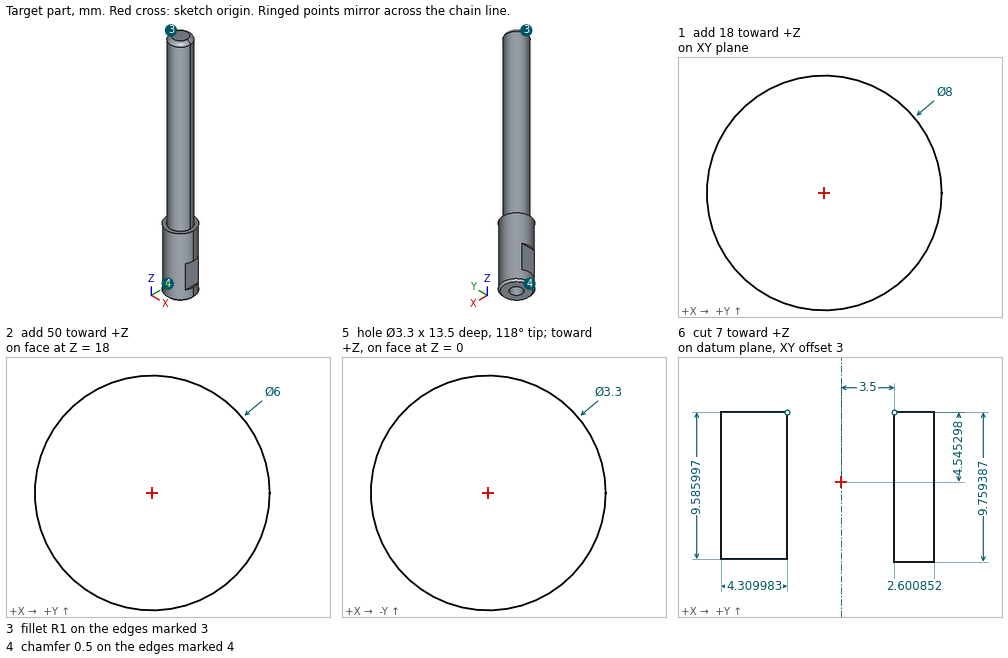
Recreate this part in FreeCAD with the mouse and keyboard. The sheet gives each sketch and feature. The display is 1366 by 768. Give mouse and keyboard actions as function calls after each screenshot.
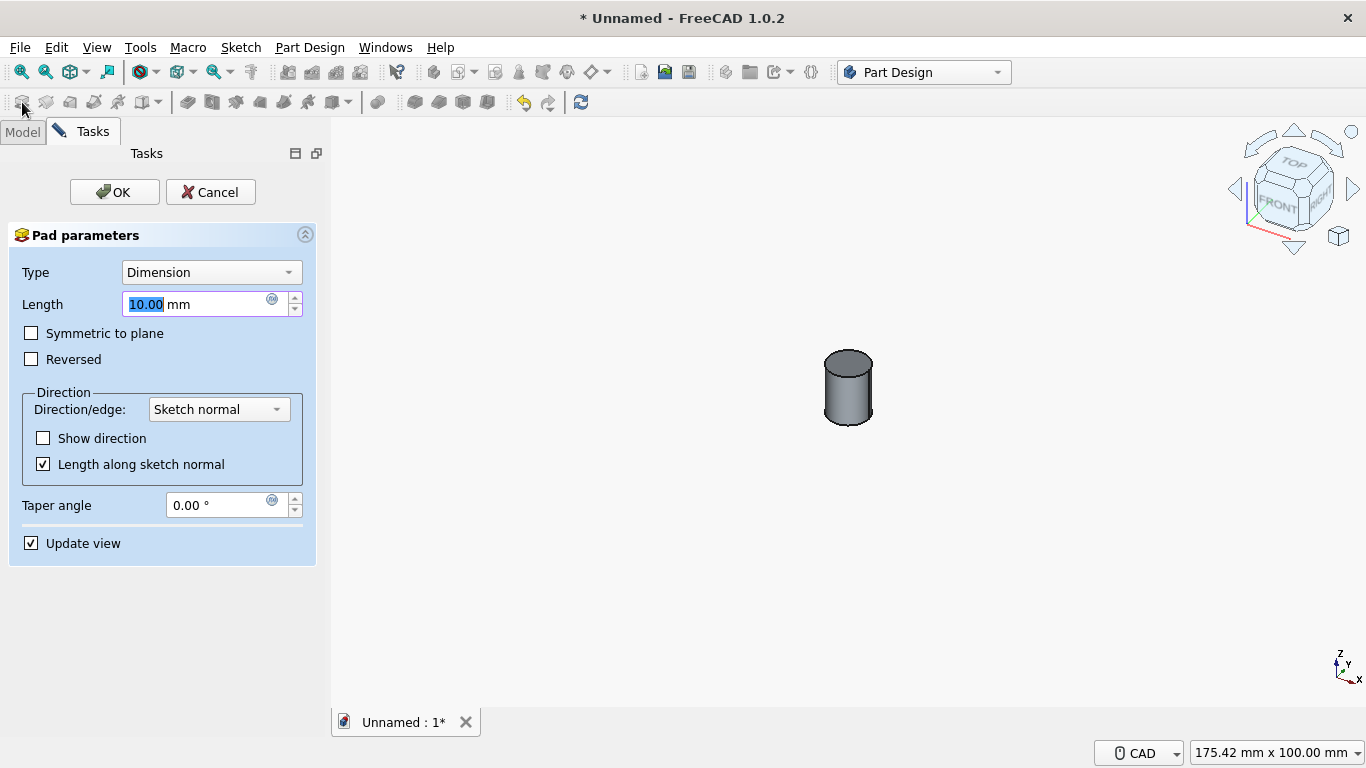
text(18)
key(Tab)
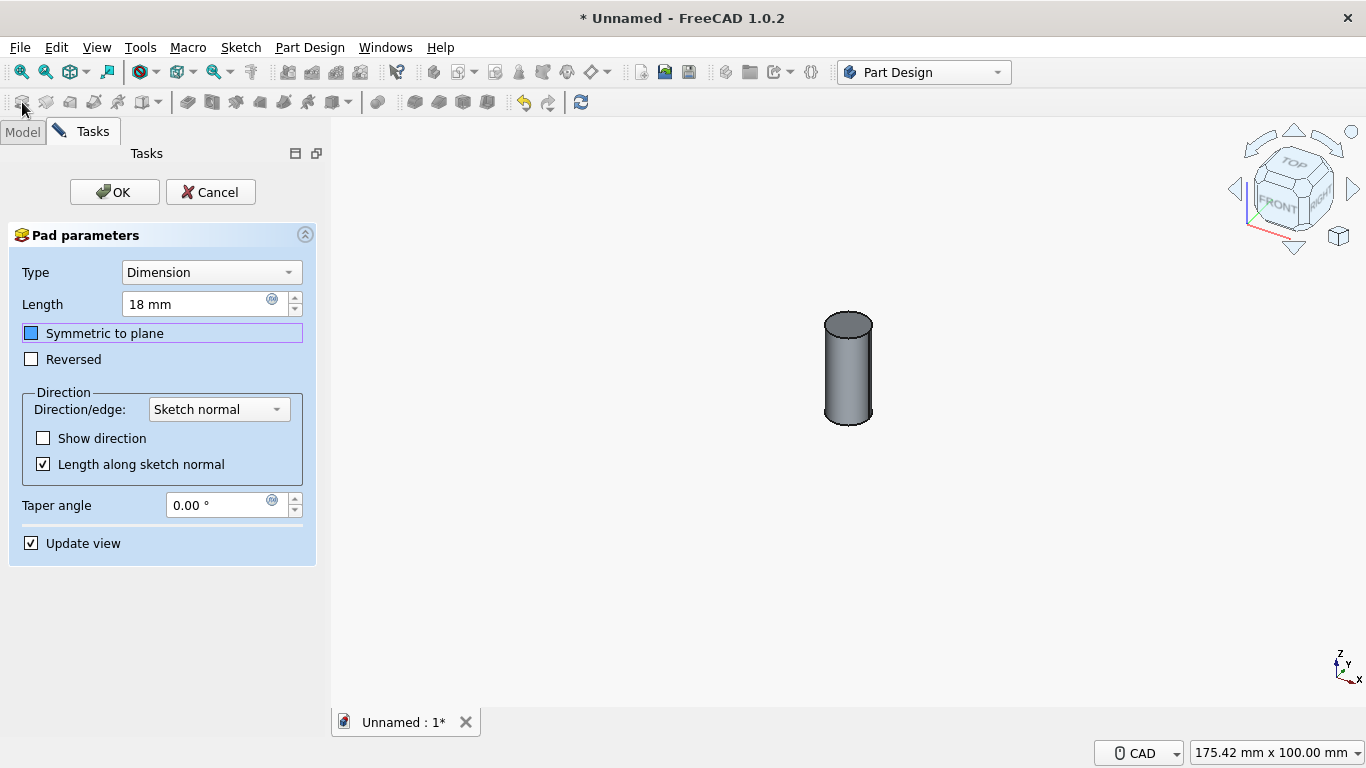
click(115, 192)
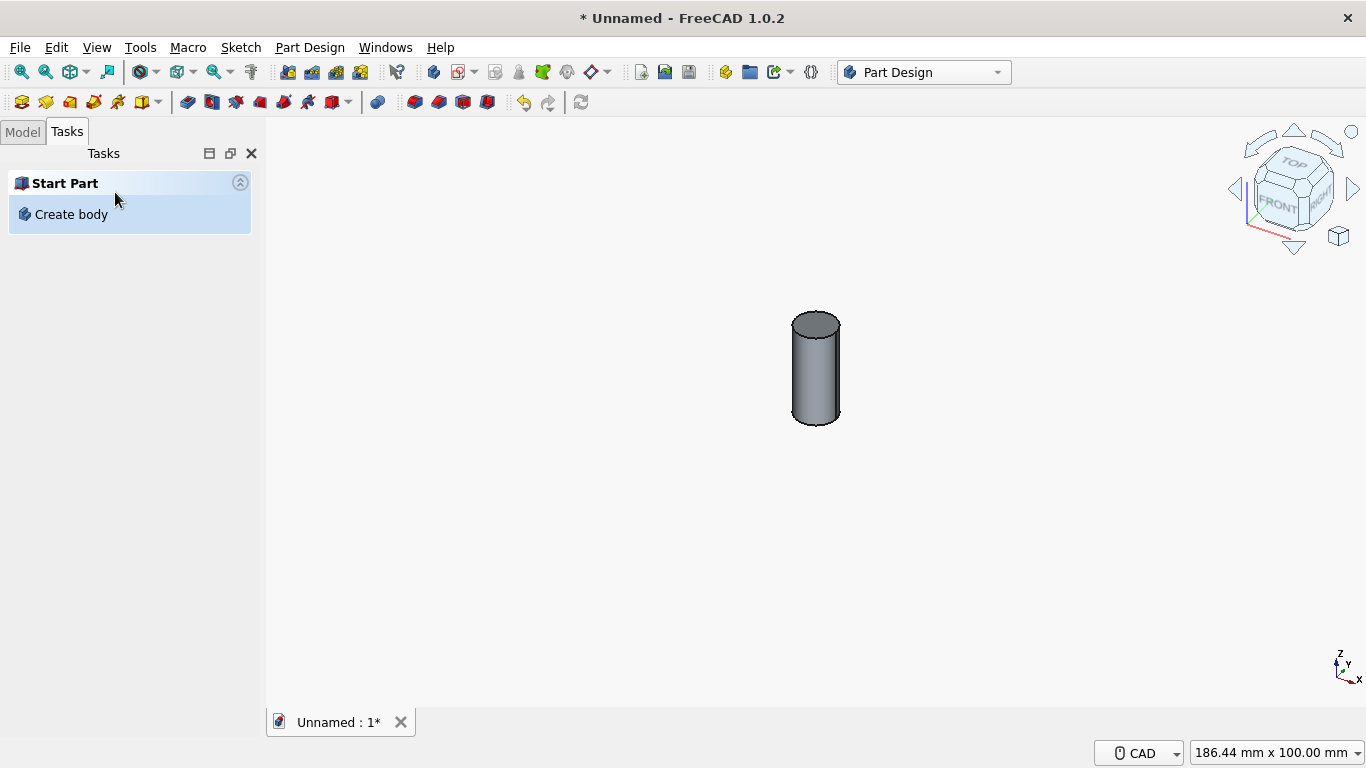
click(22, 72)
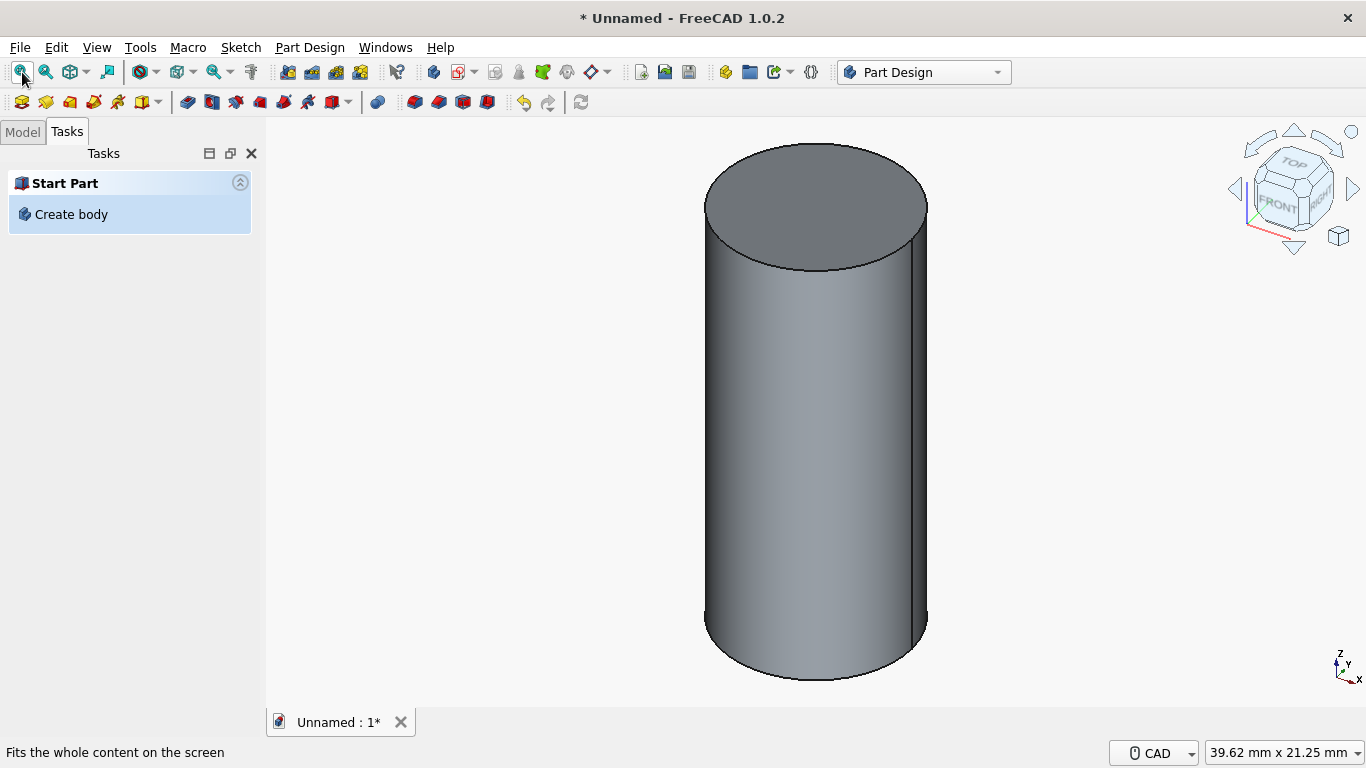
click(816, 206)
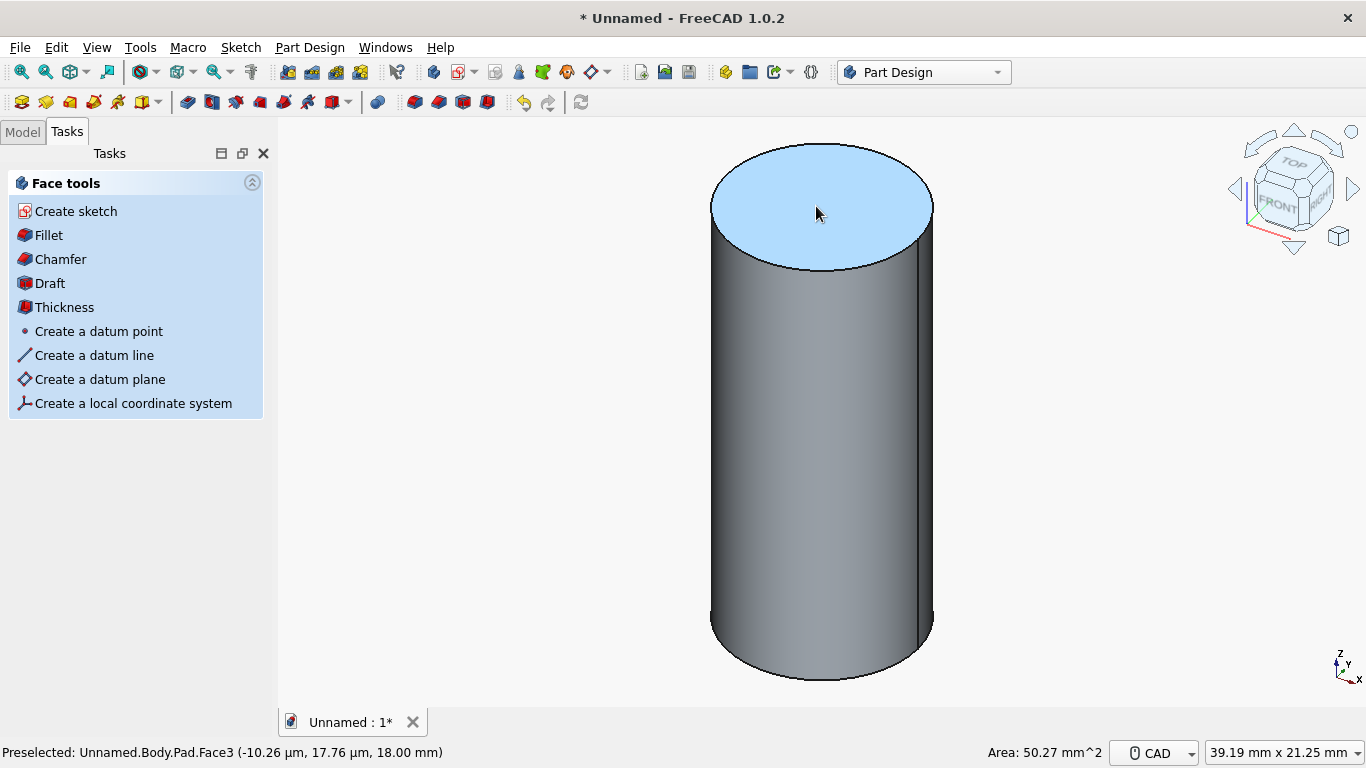
click(458, 72)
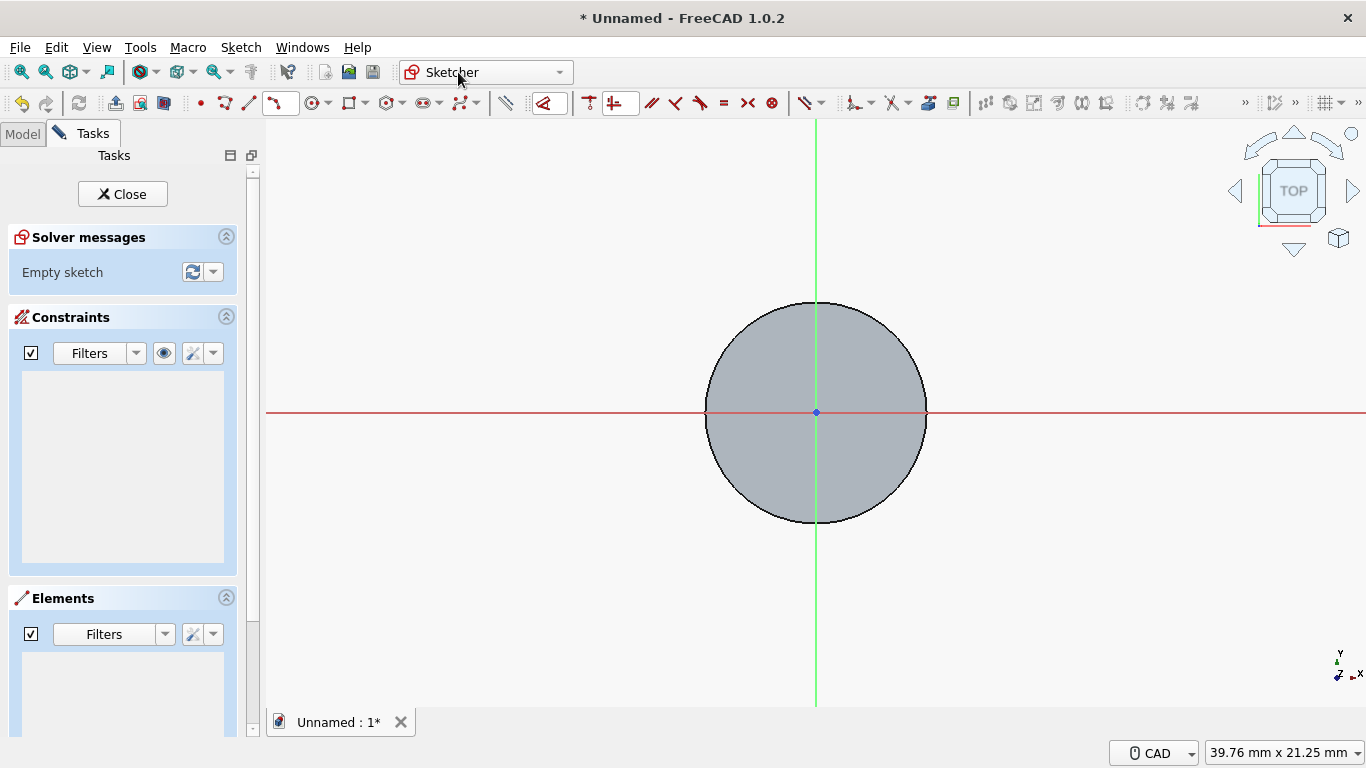
scroll(872, 413, up, 4)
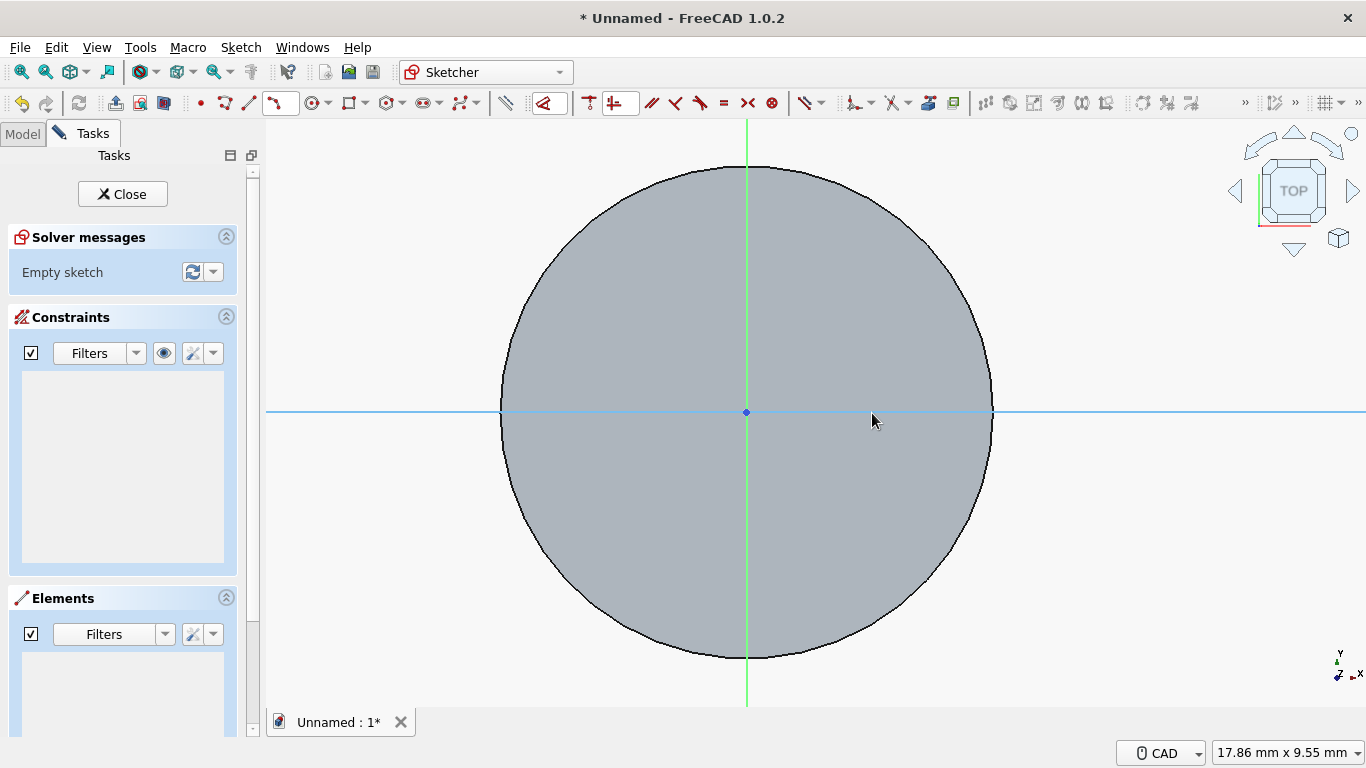
click(312, 104)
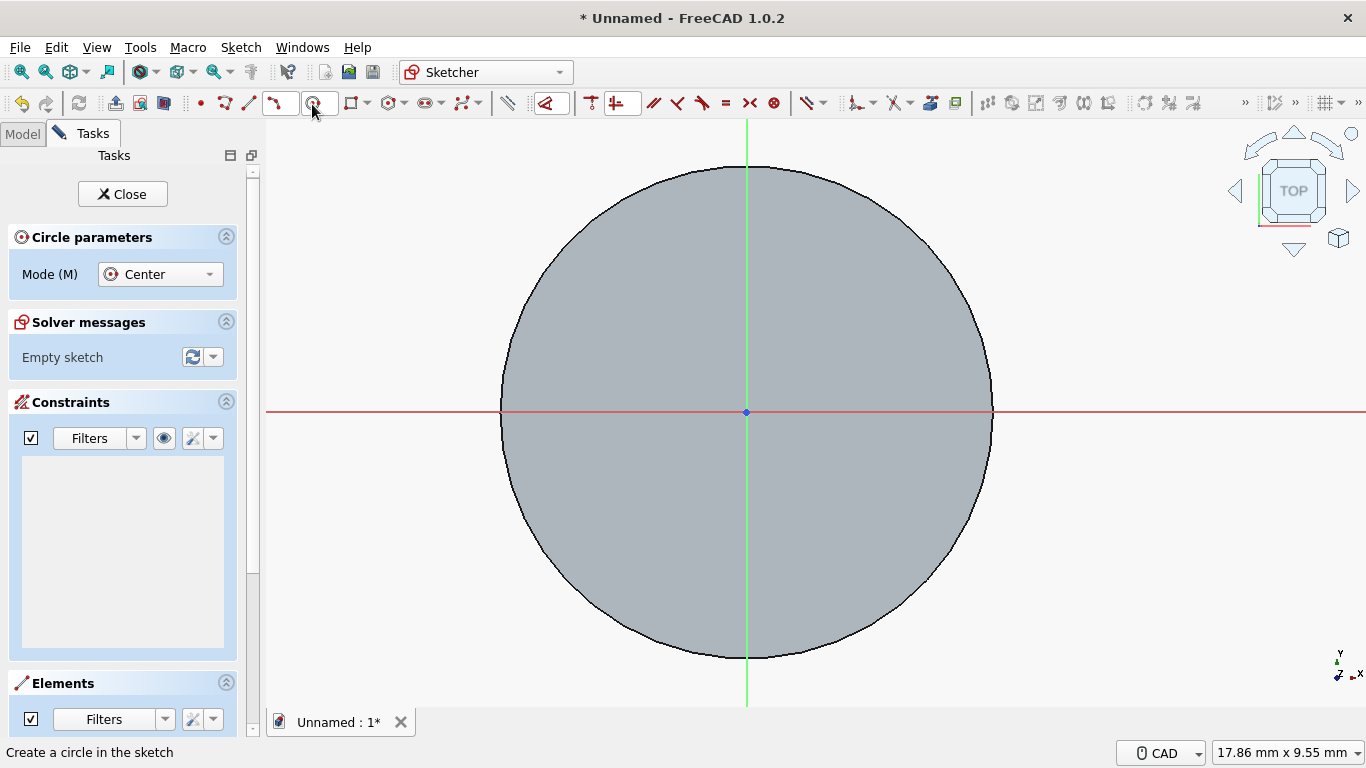
click(747, 412)
move(877, 282)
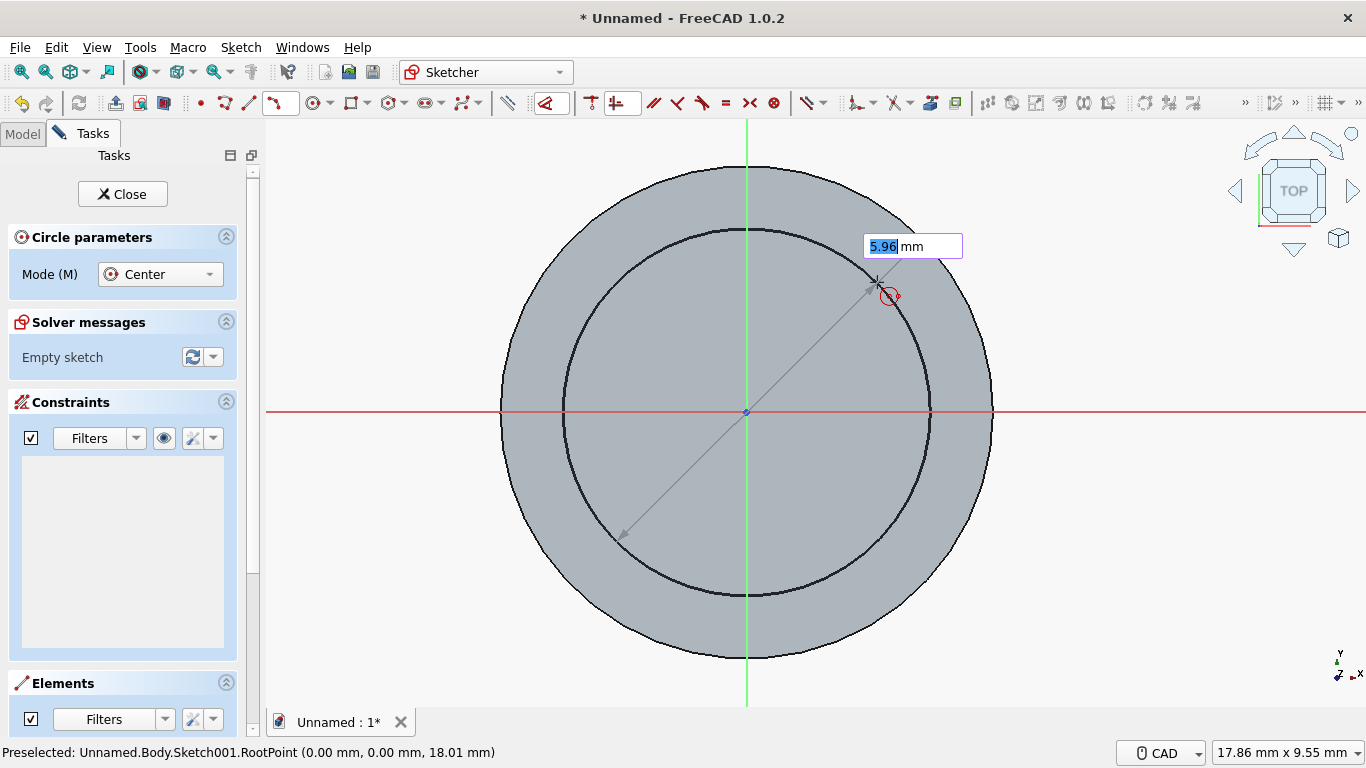
text(6)
key(Return)
key(Escape)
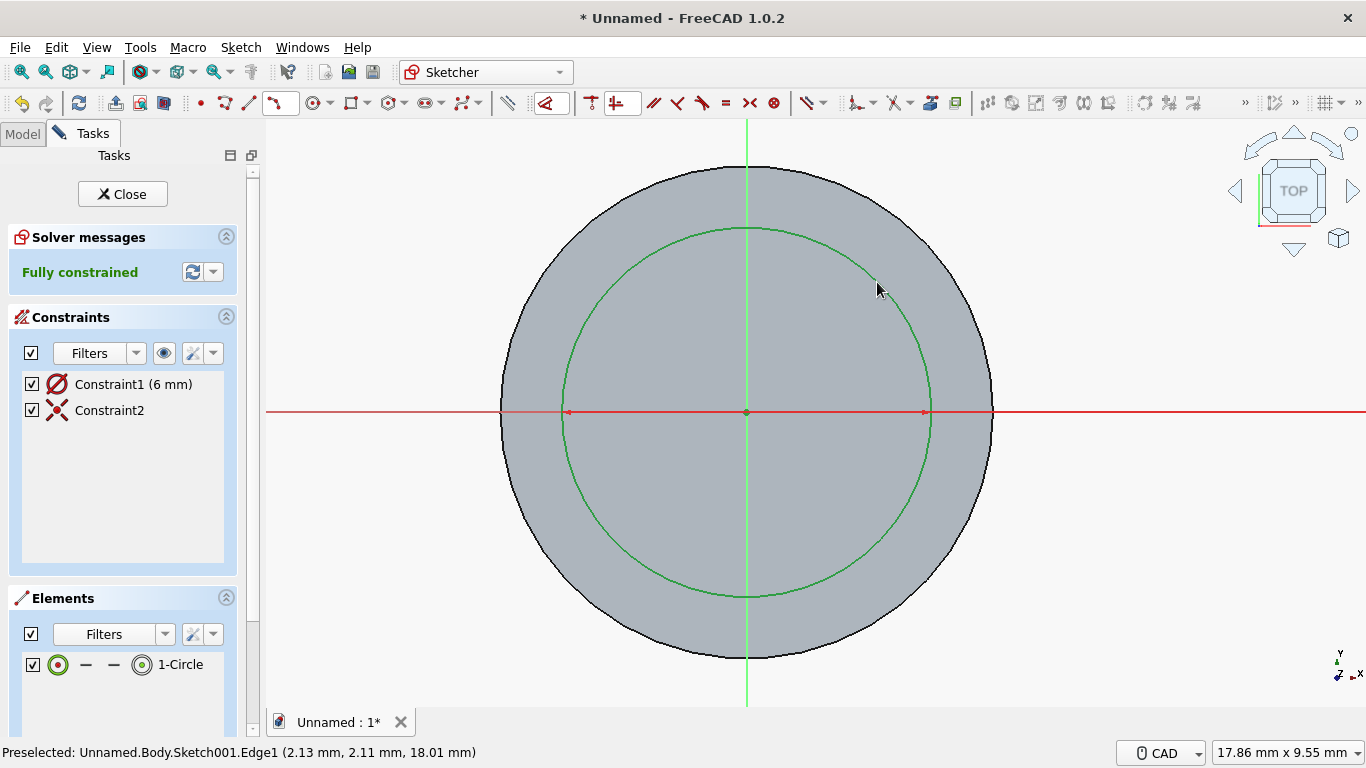
click(123, 194)